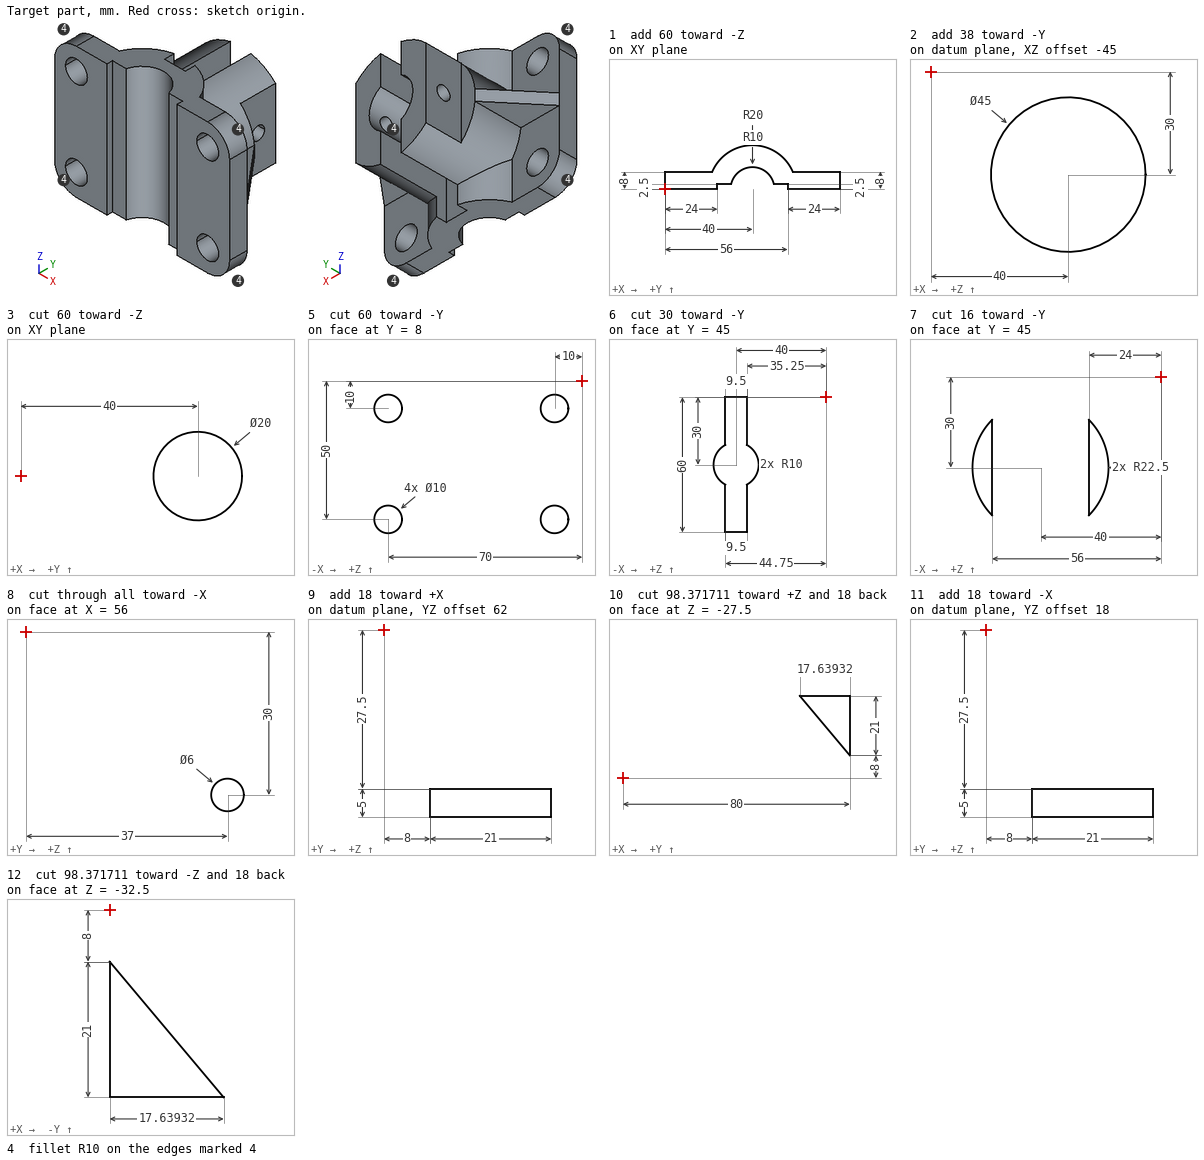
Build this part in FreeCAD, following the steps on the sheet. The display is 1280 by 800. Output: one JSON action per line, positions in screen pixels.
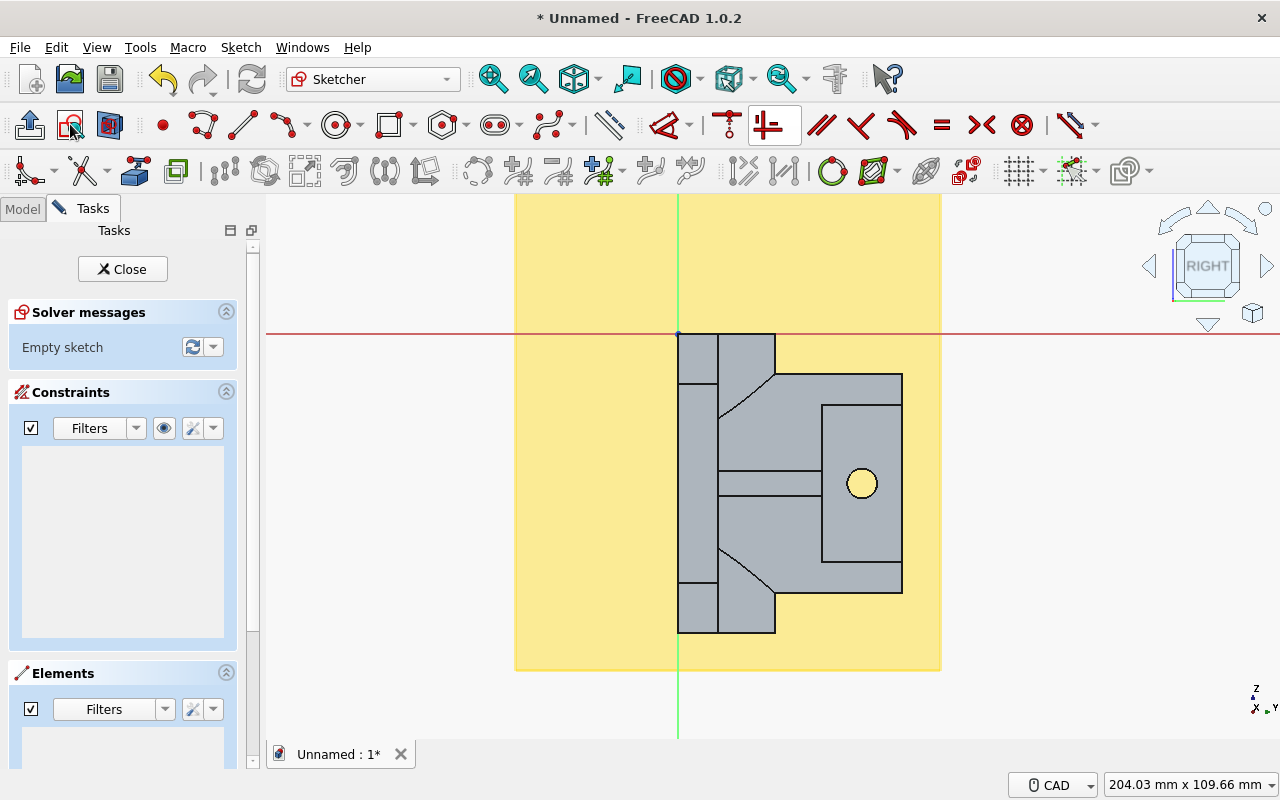
{"action": "left_click", "coordinate": [110, 126]}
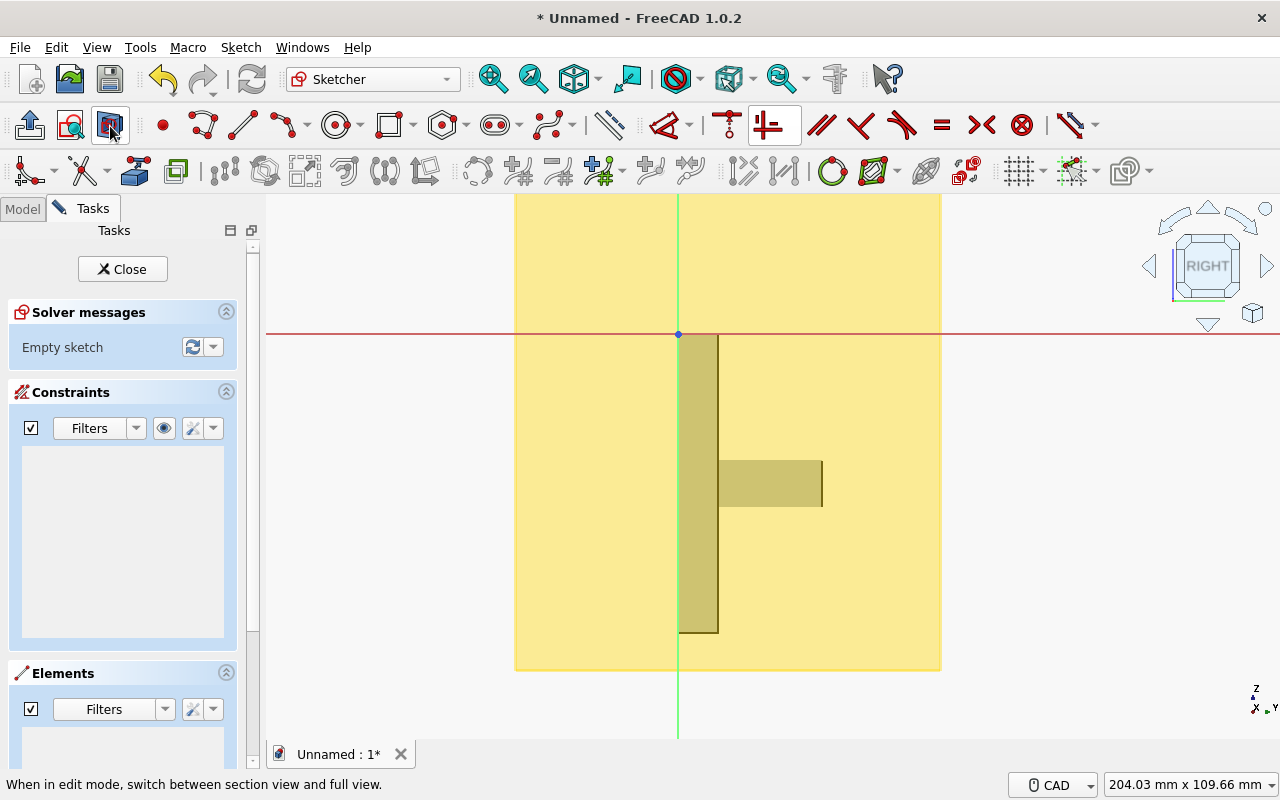
{"action": "scroll", "coordinate": [788, 373], "scroll_direction": "up", "scroll_amount": 4}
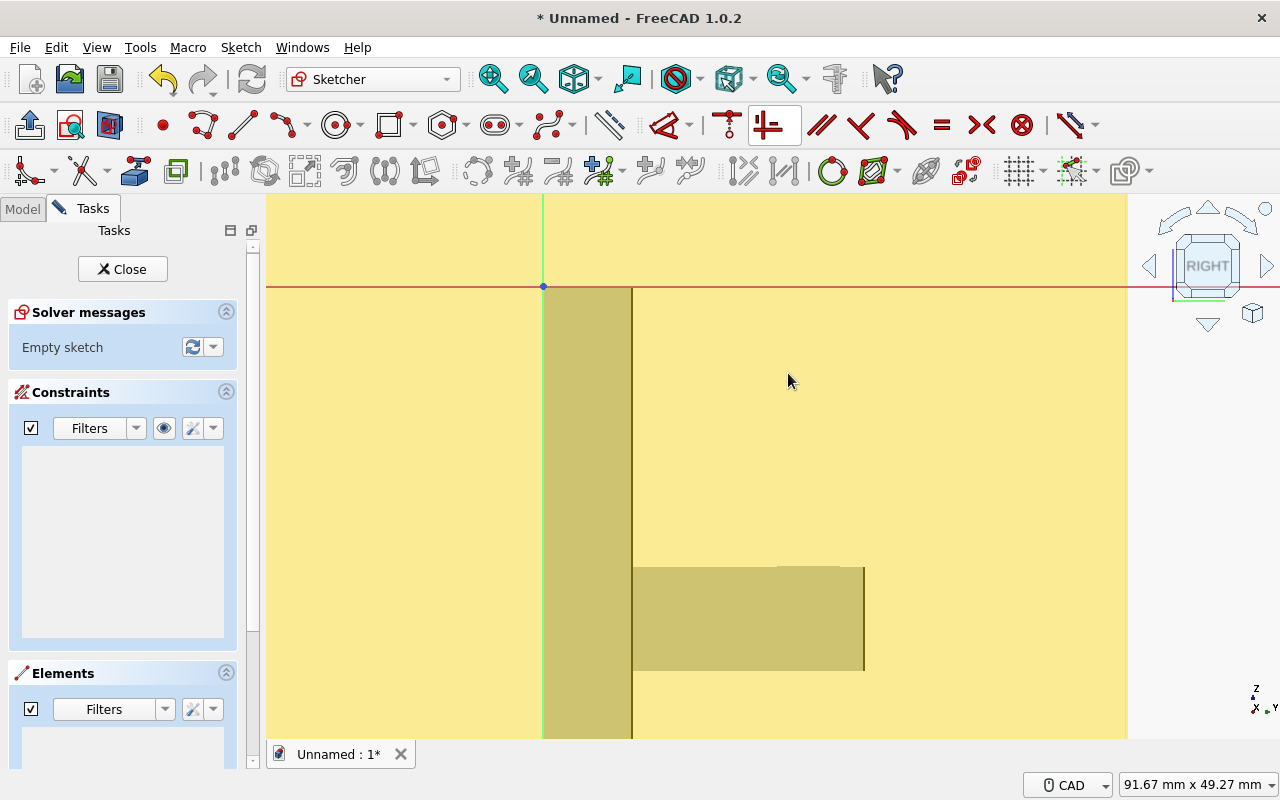
{"action": "left_click", "coordinate": [390, 126]}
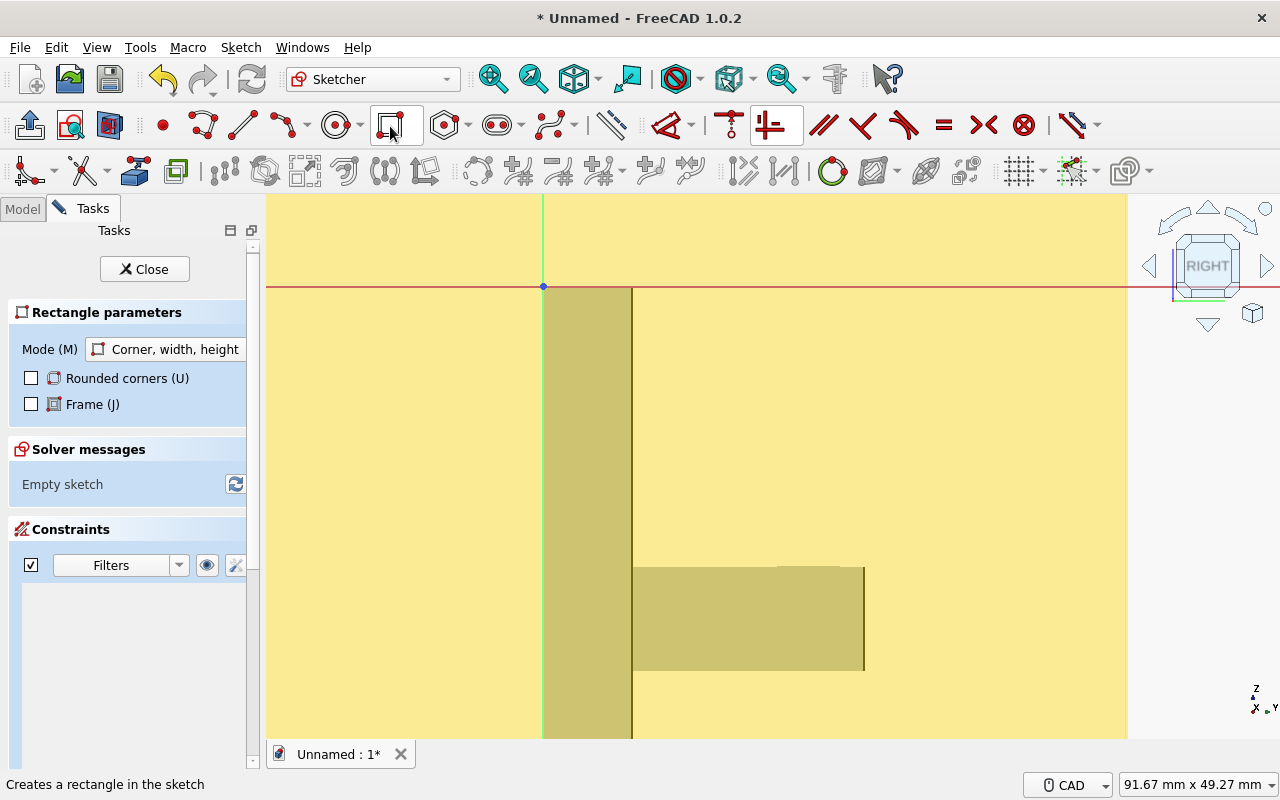
{"action": "left_click", "coordinate": [632, 591]}
{"action": "left_click", "coordinate": [864, 646]}
{"action": "key", "text": "Escape"}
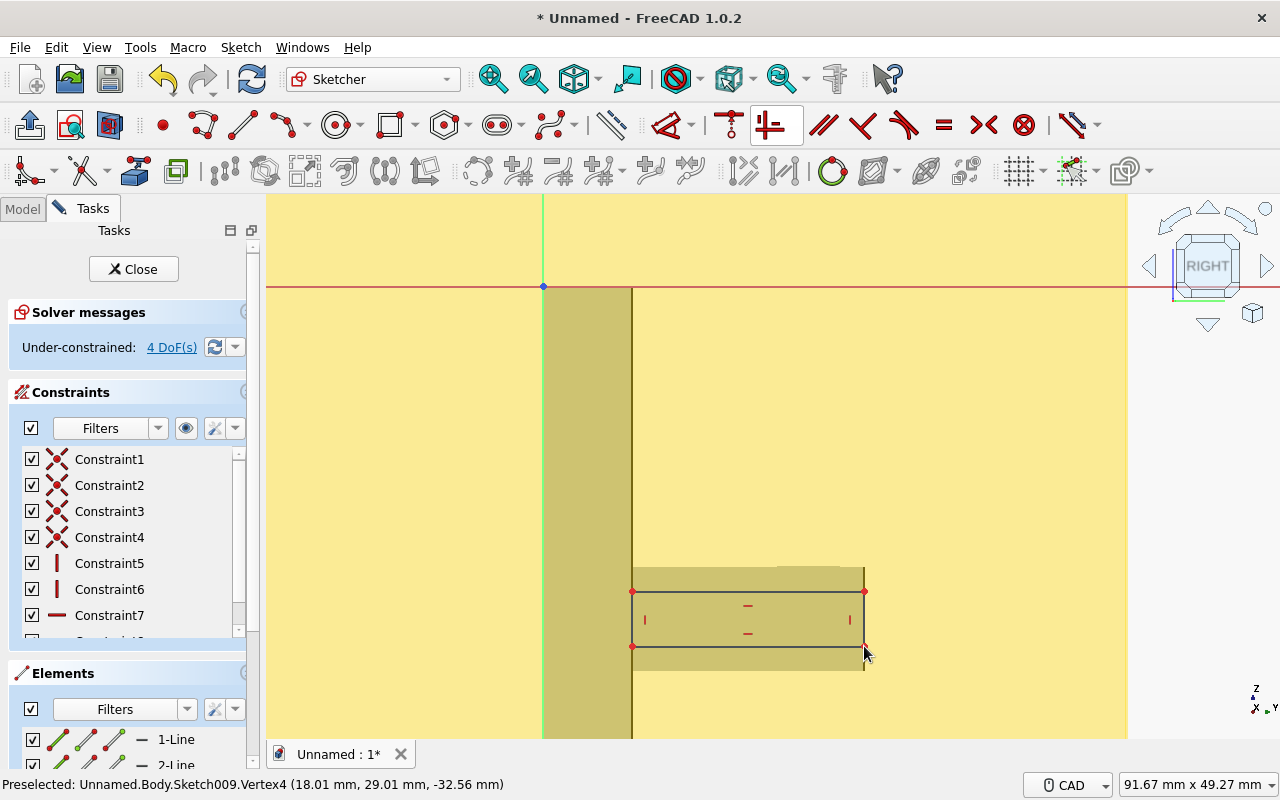
{"action": "left_click", "coordinate": [666, 126]}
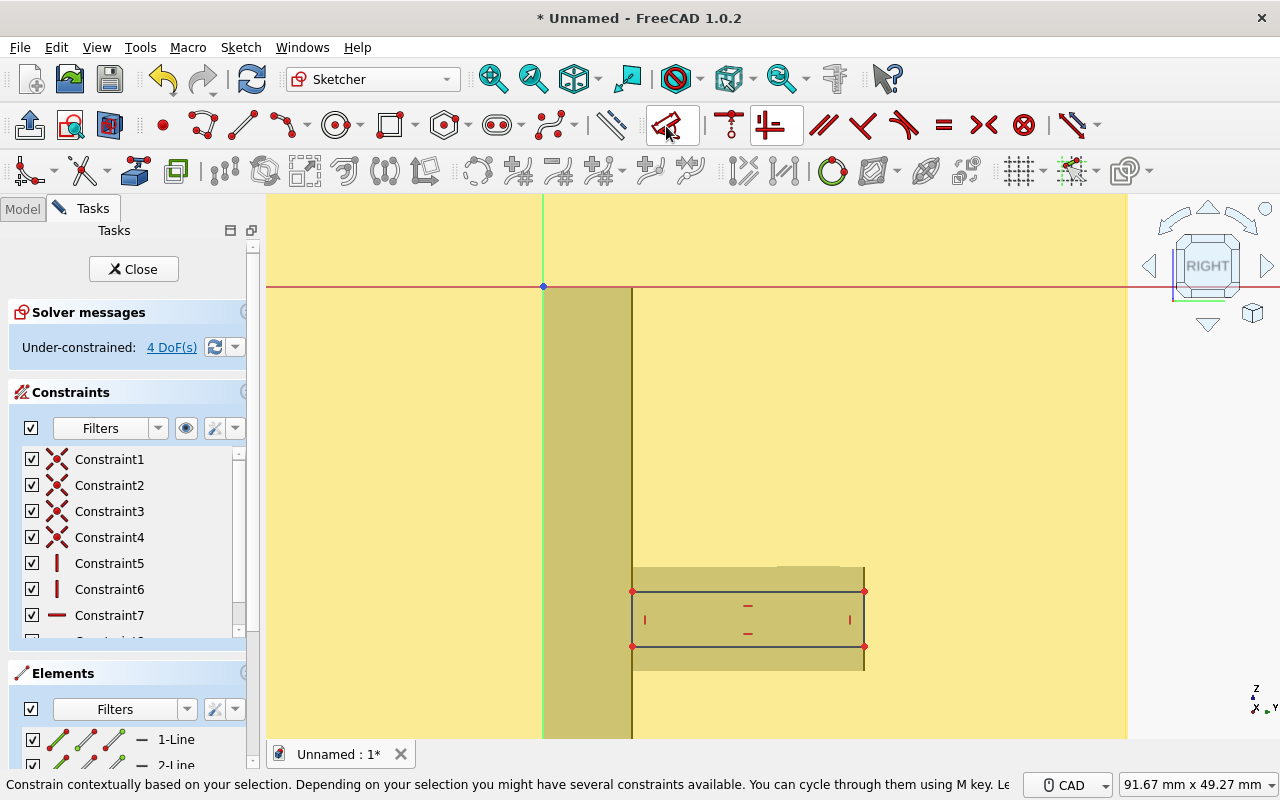
{"action": "left_click", "coordinate": [632, 608]}
{"action": "left_click", "coordinate": [598, 619]}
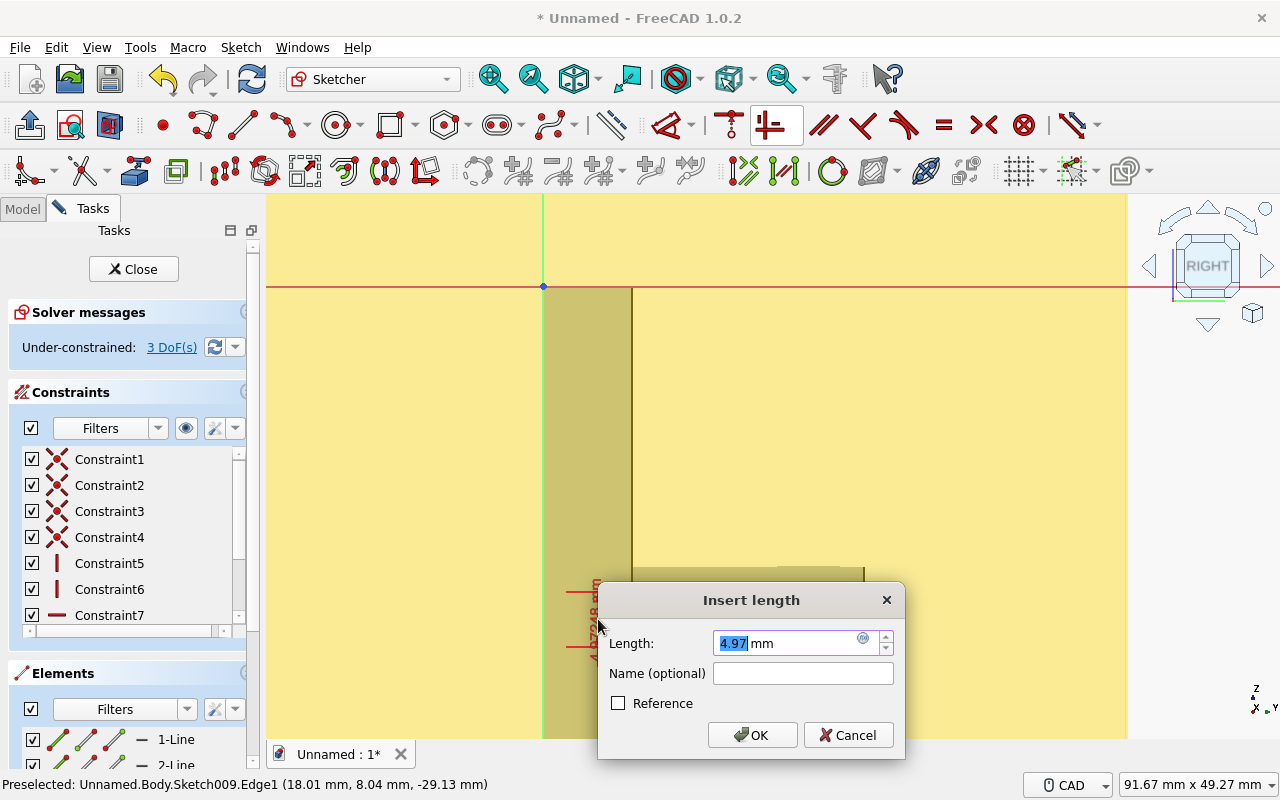
{"action": "type", "text": "5"}
{"action": "key", "text": "Return"}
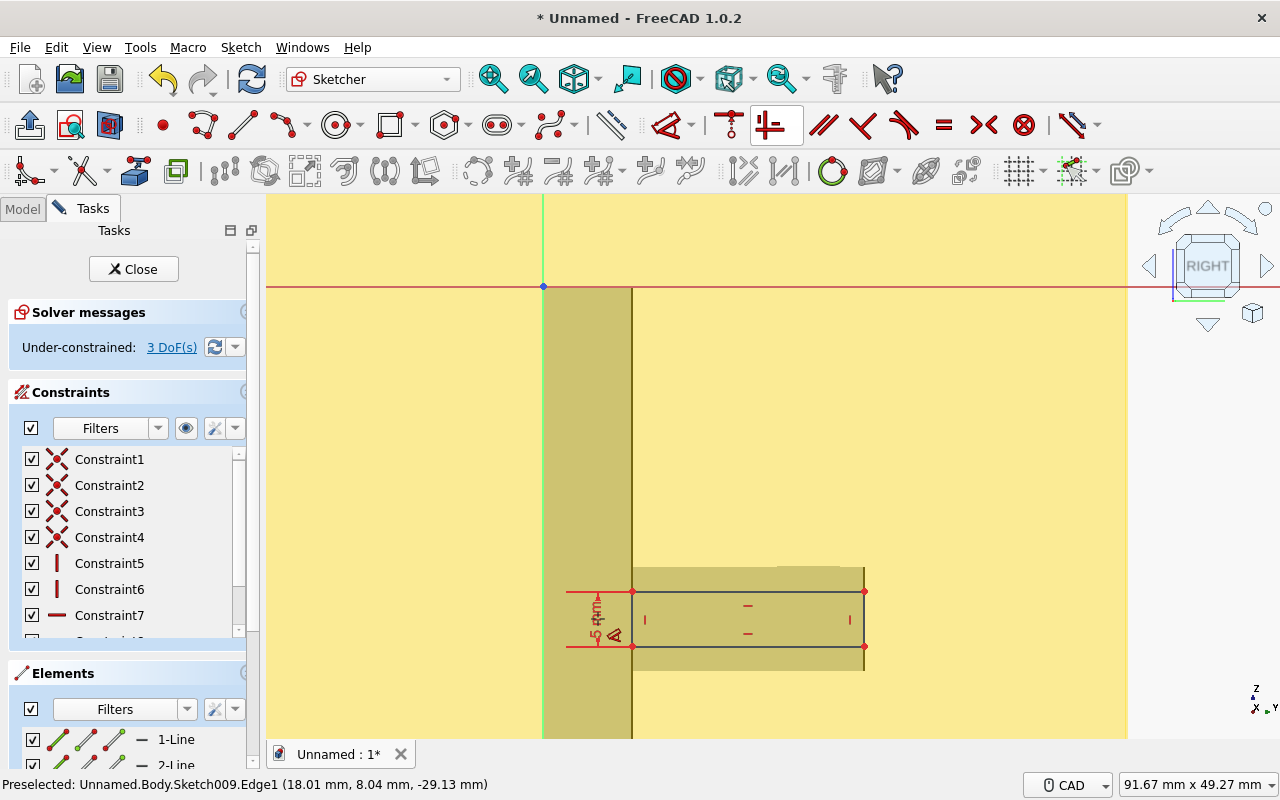
{"action": "left_click", "coordinate": [702, 647]}
{"action": "left_click", "coordinate": [748, 681]}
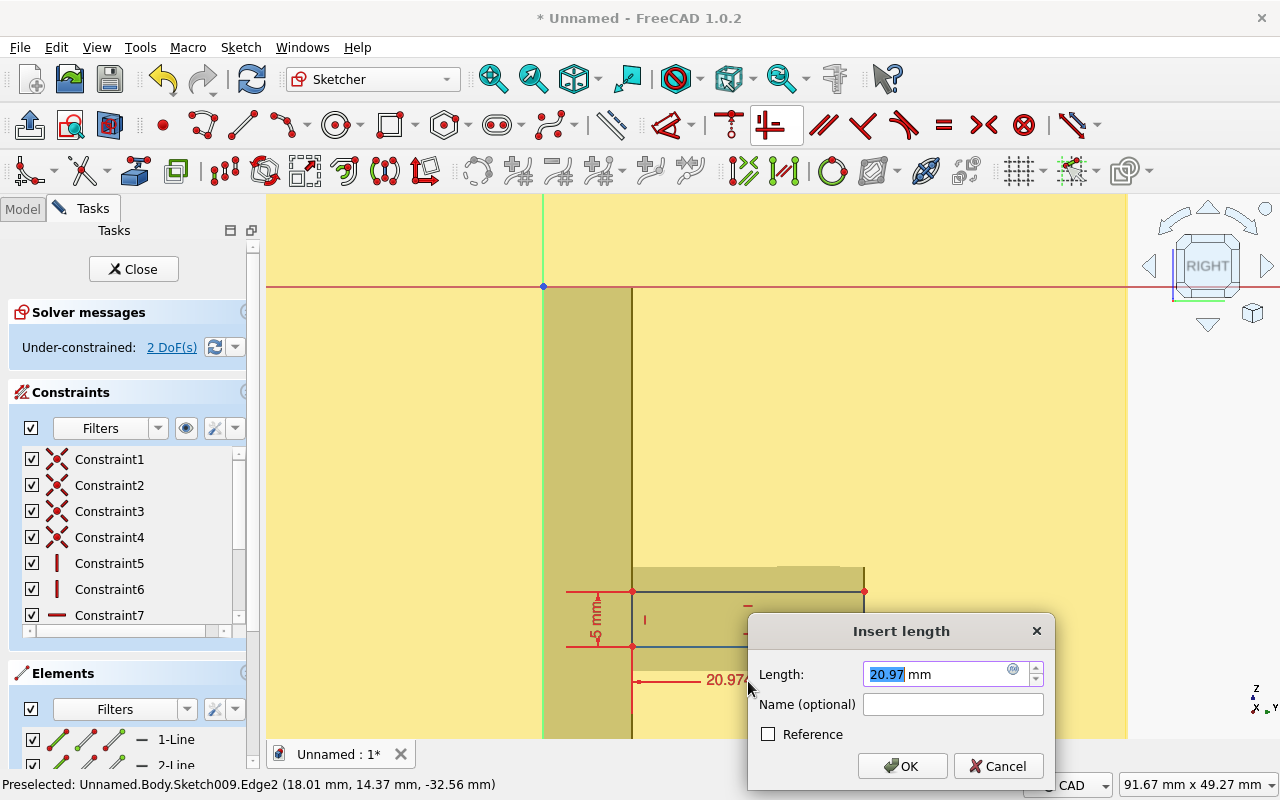
{"action": "type", "text": "21"}
{"action": "key", "text": "Return"}